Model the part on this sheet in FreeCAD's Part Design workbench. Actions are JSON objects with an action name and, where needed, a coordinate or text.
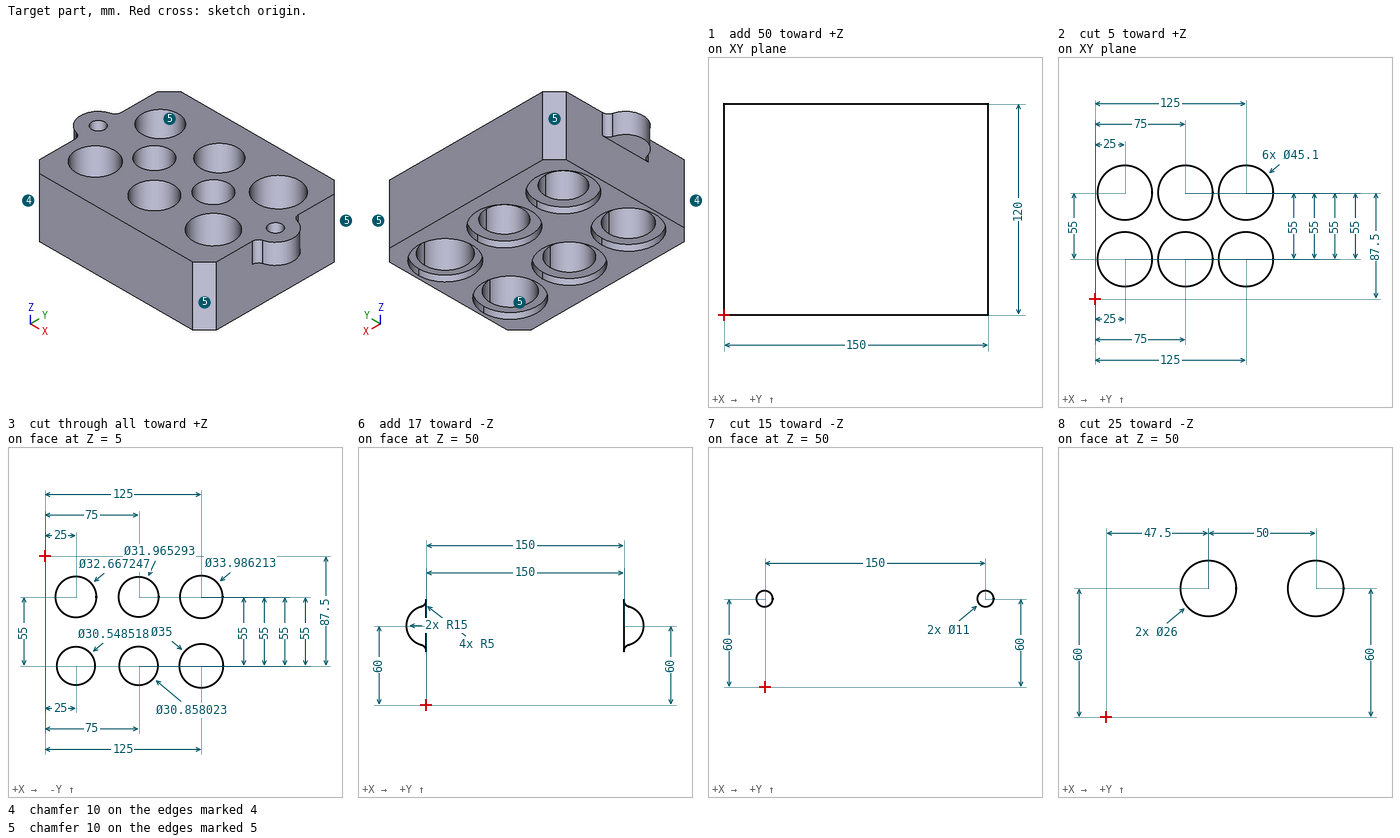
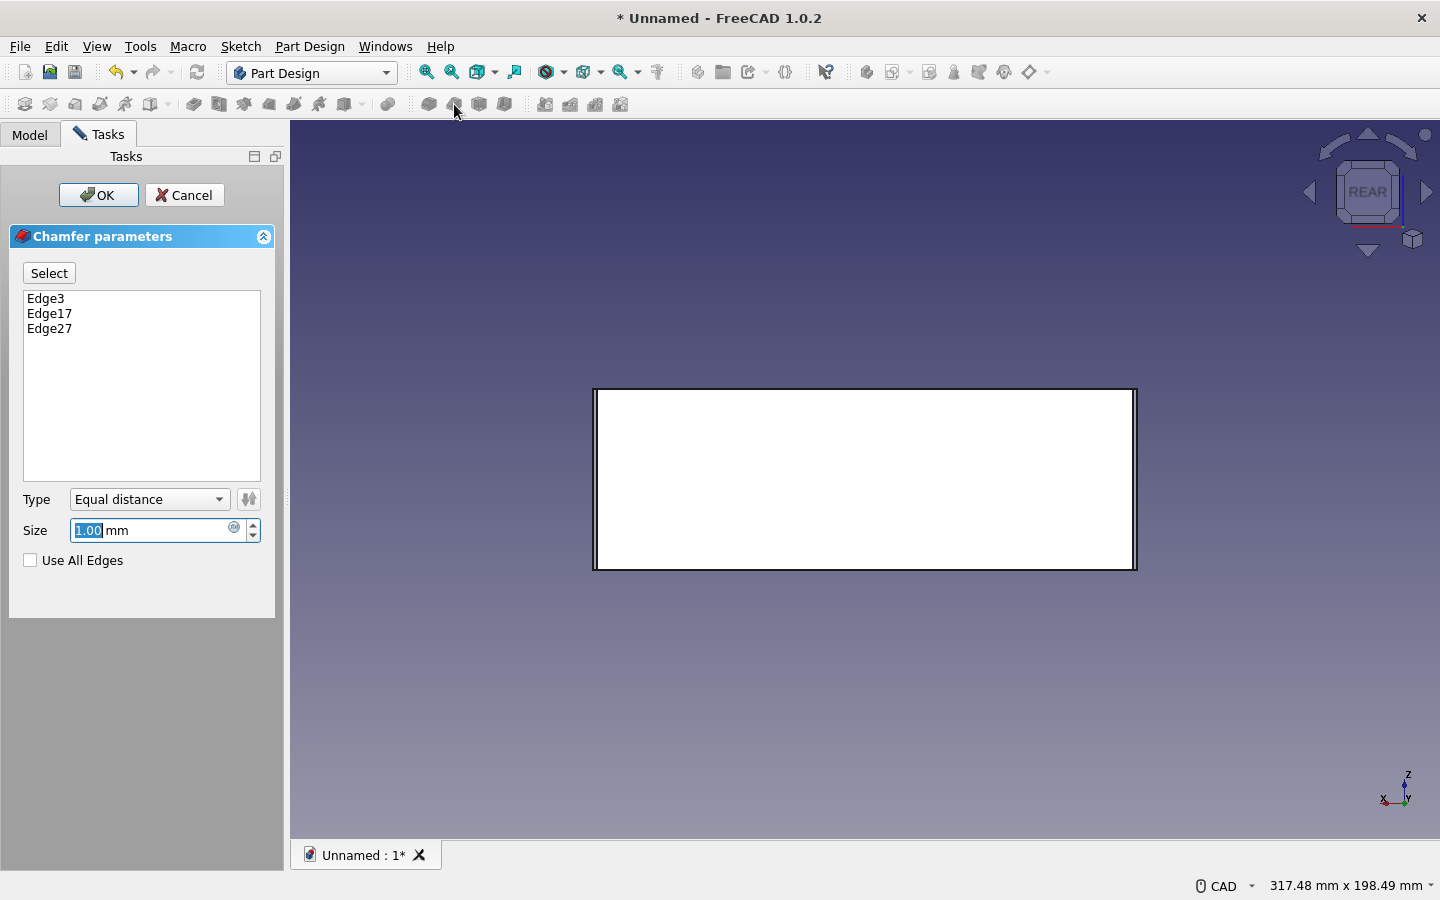
{"action": "type", "text": "10"}
{"action": "key", "text": "Tab"}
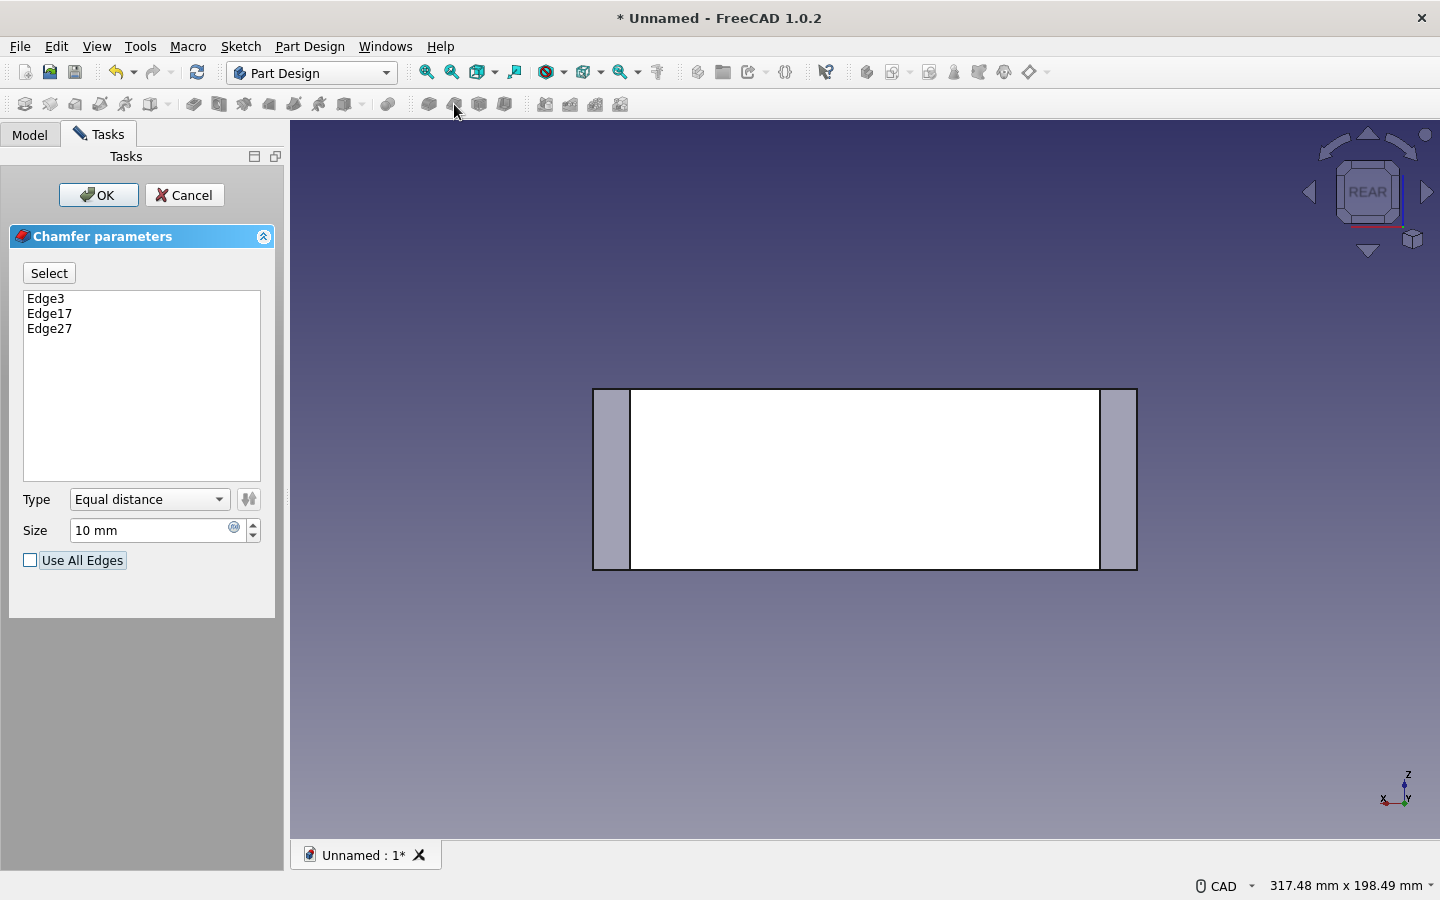
{"action": "left_click", "coordinate": [99, 195]}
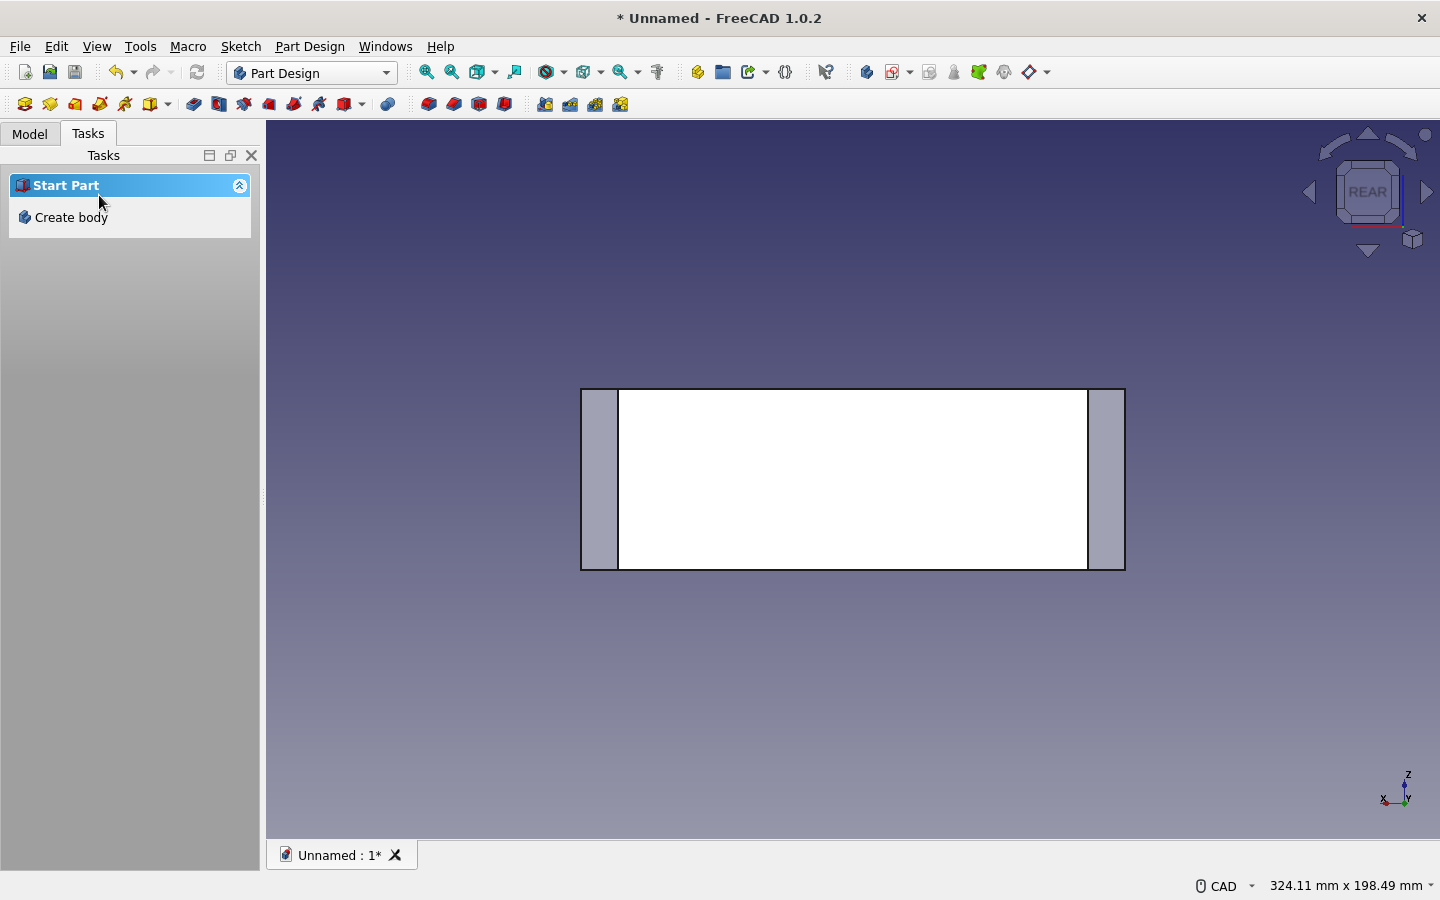
{"action": "key", "text": "0"}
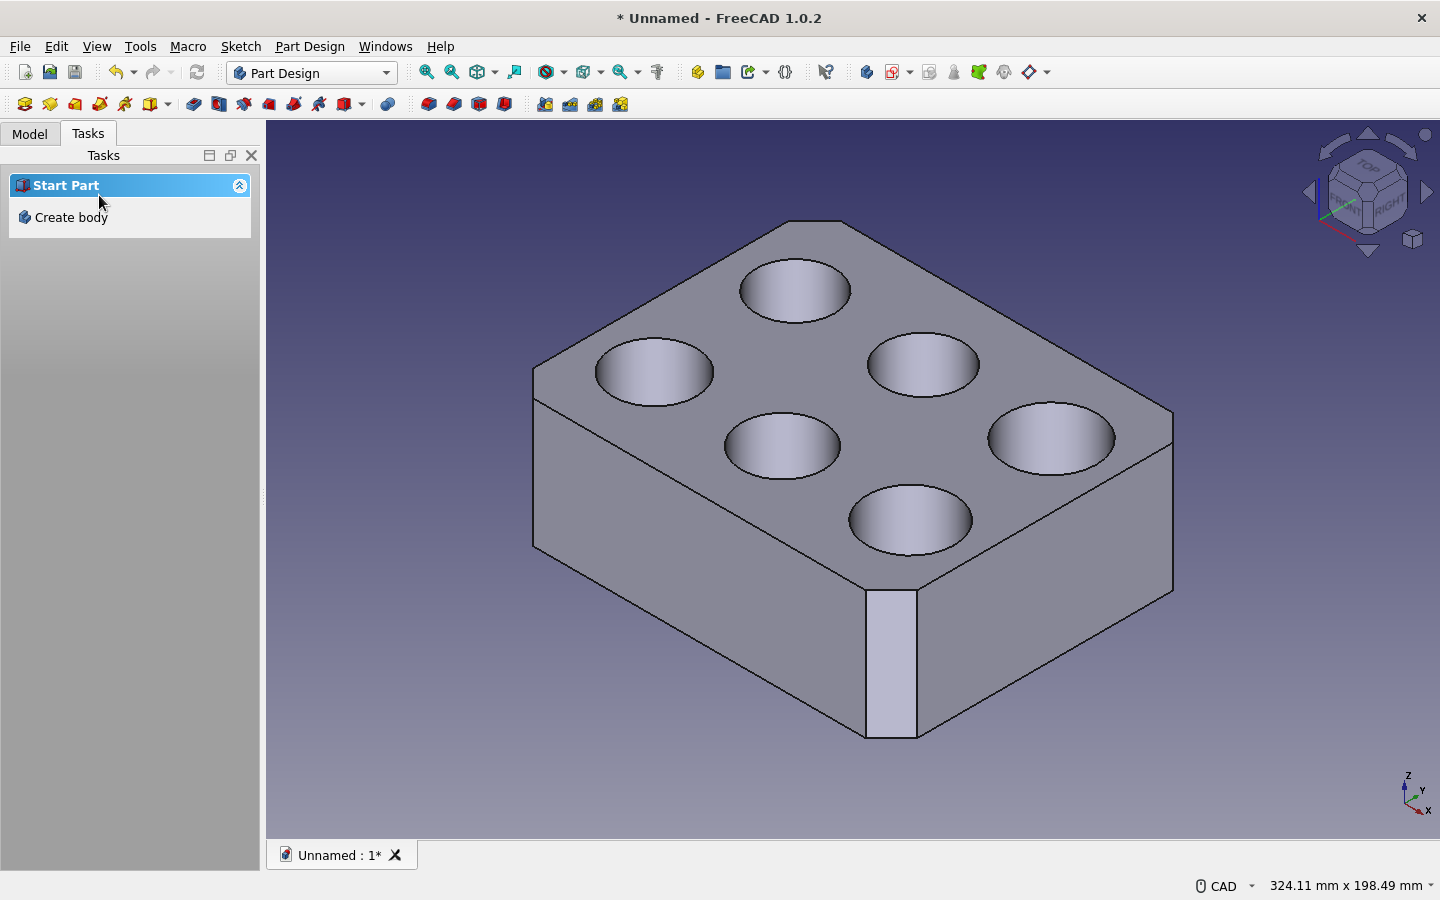
{"action": "left_click", "coordinate": [908, 436]}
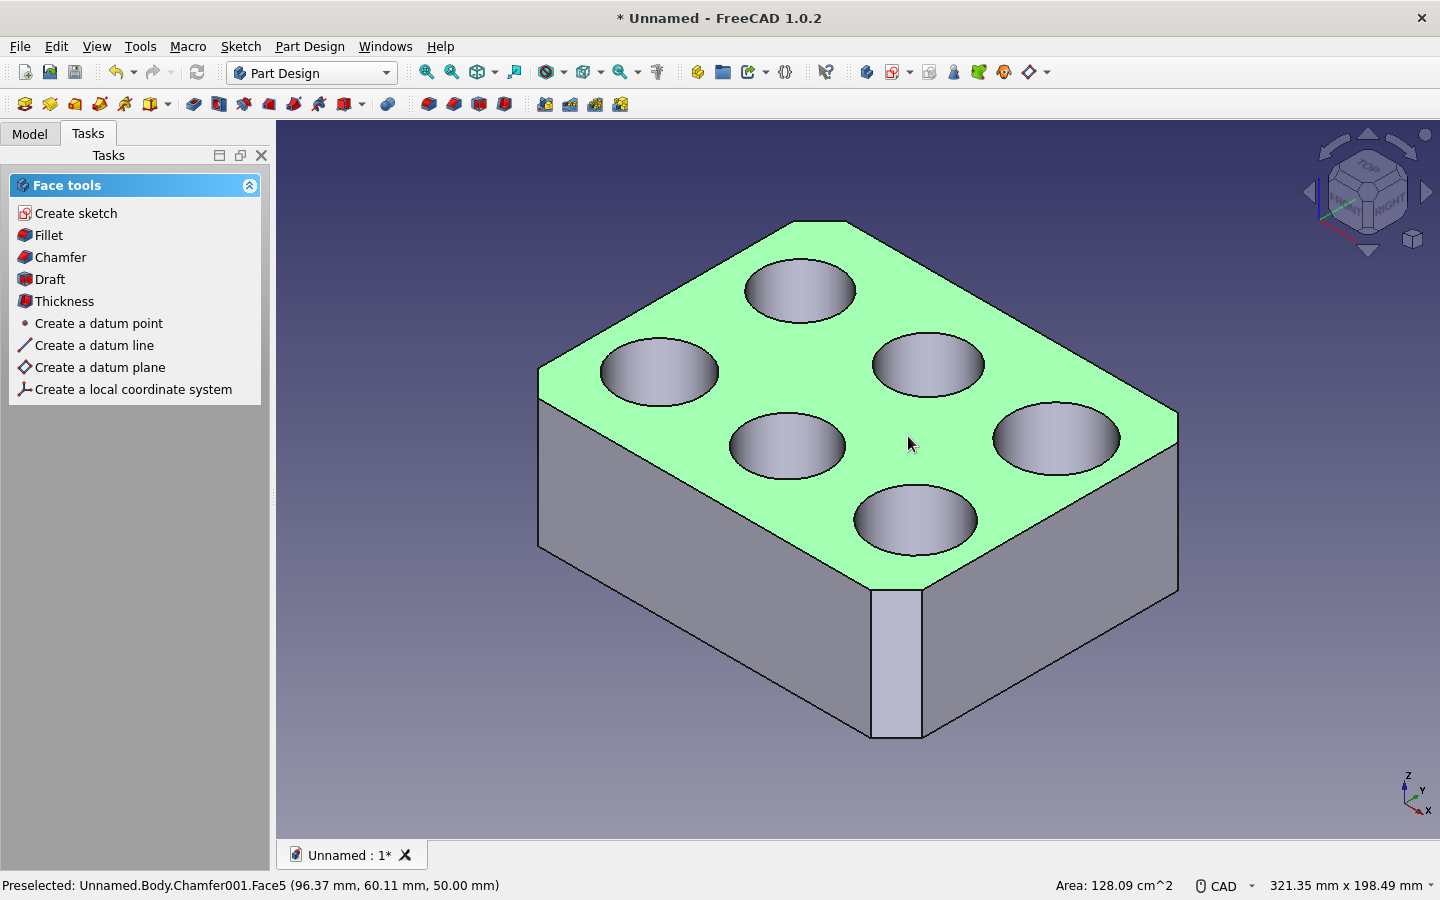
{"action": "left_click", "coordinate": [892, 72]}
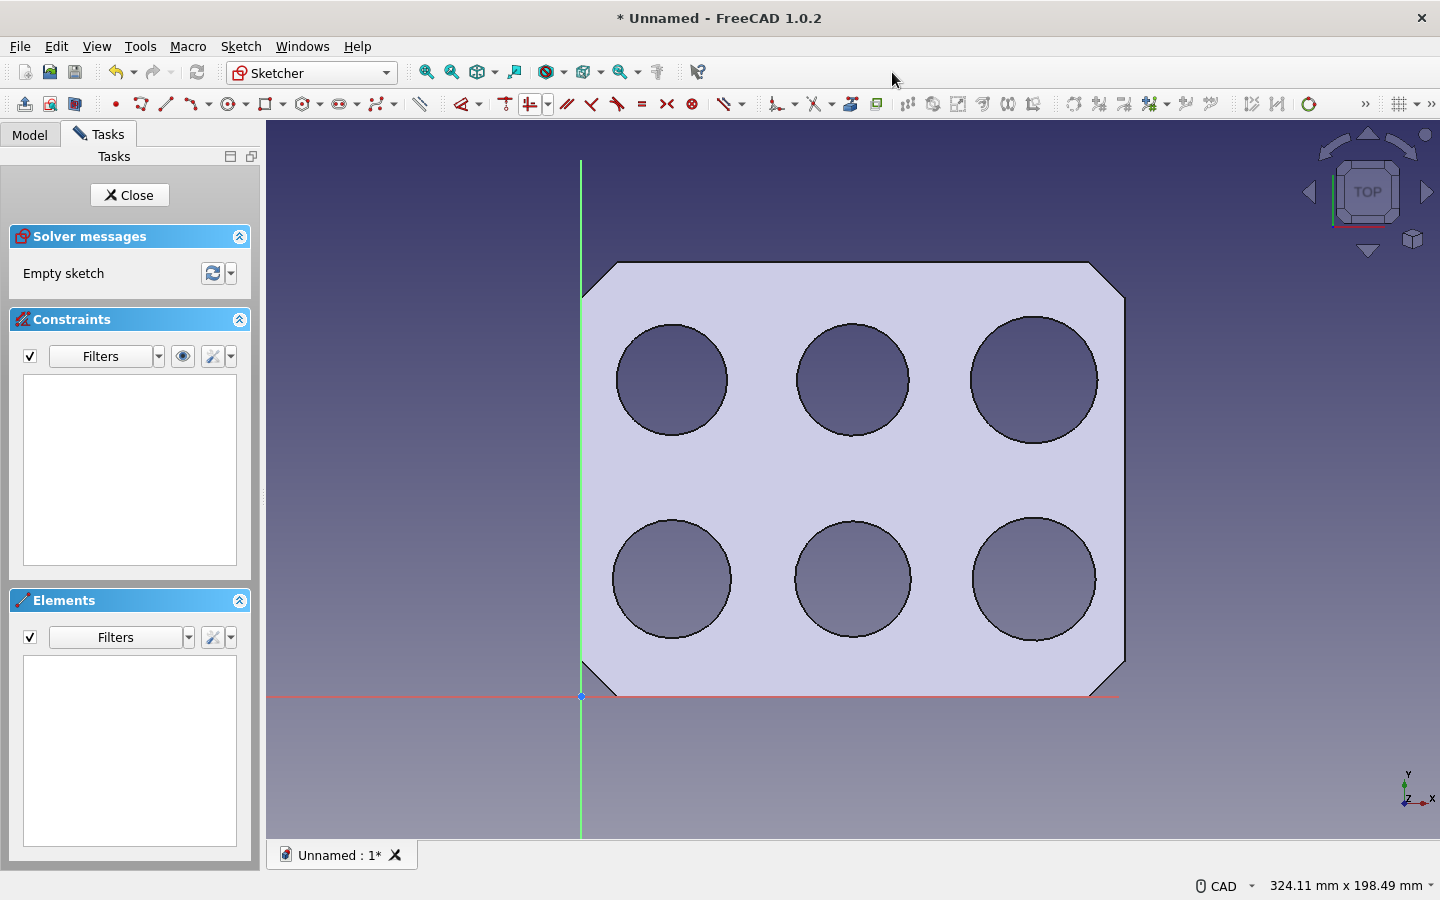
{"action": "left_click", "coordinate": [166, 104]}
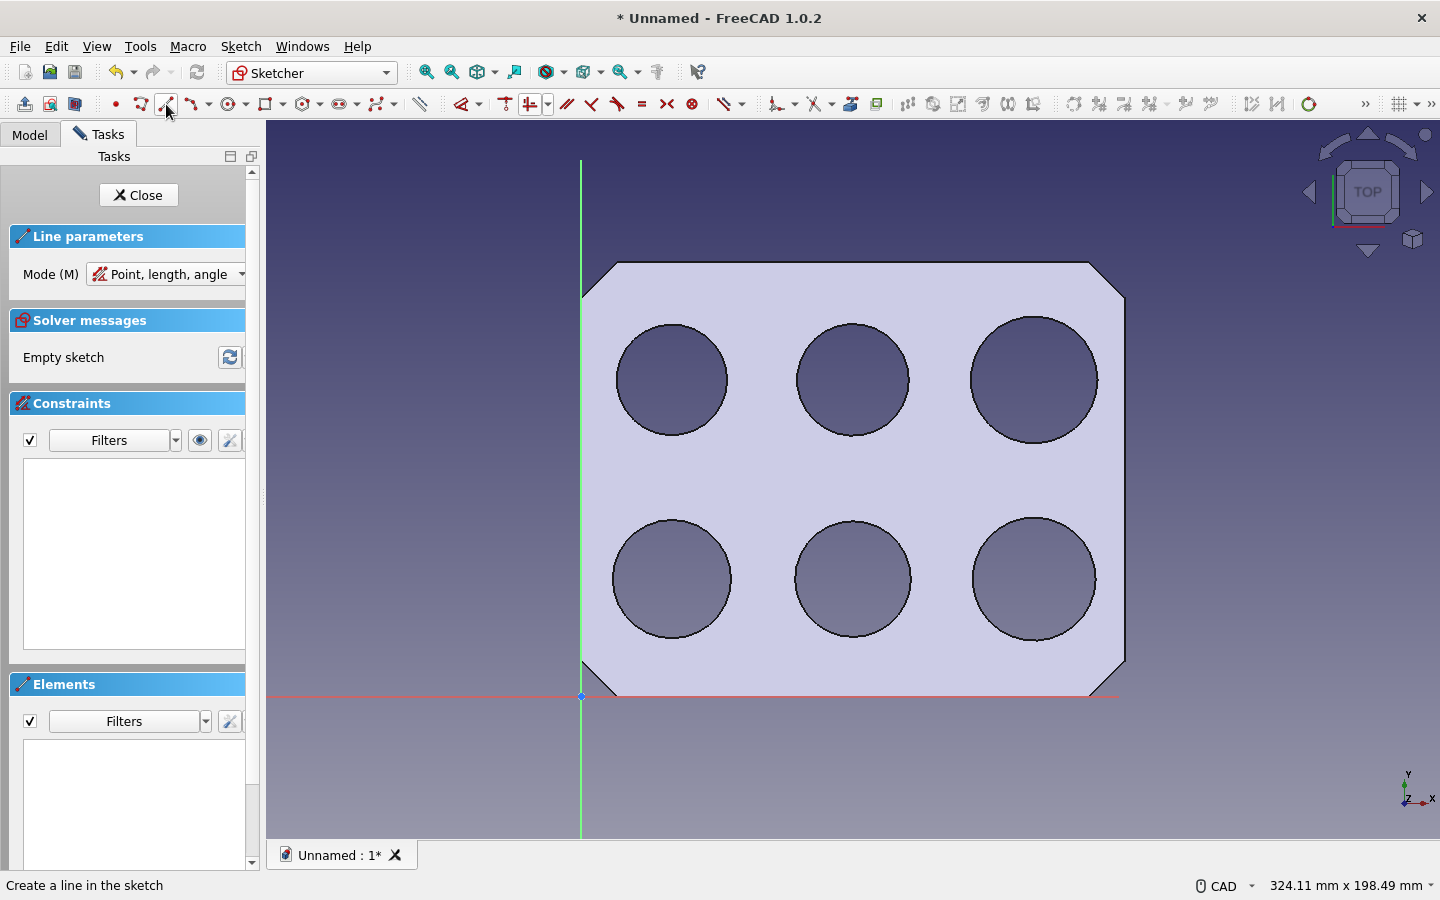
{"action": "left_click", "coordinate": [581, 550]}
{"action": "left_click", "coordinate": [590, 409]}